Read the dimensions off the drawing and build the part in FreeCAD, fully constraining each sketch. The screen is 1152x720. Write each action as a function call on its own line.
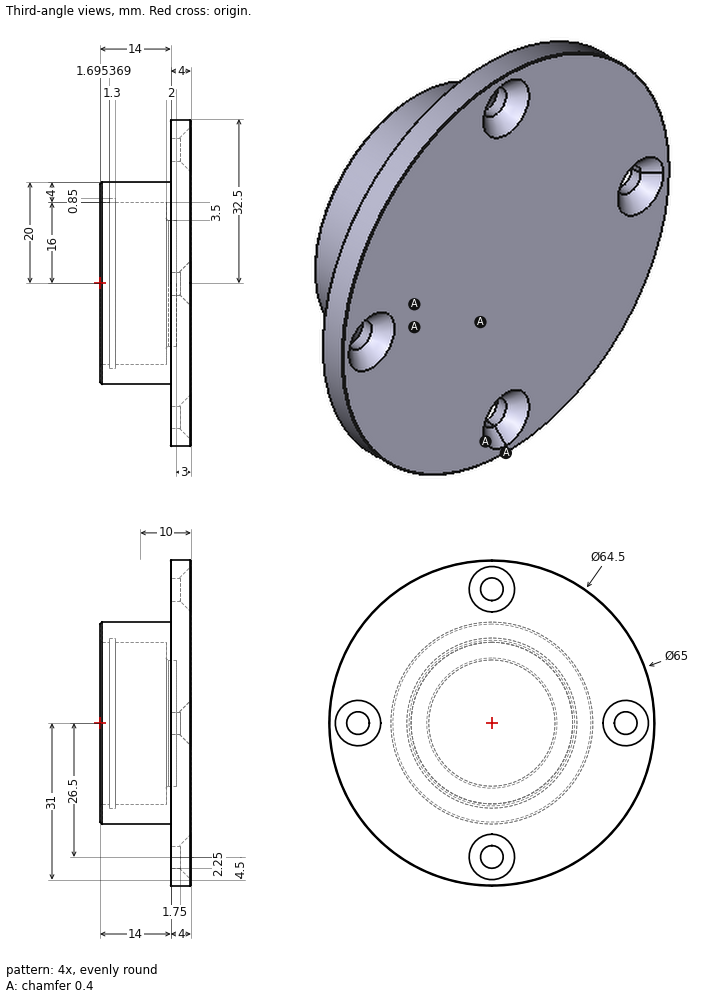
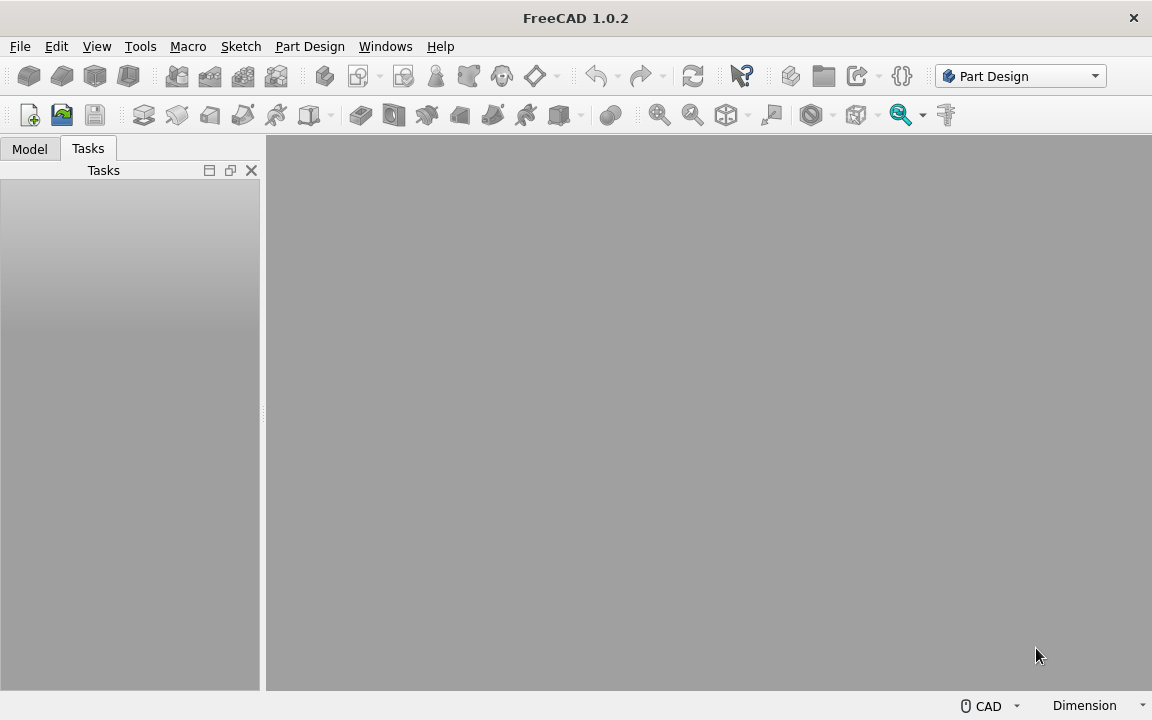
click(29, 116)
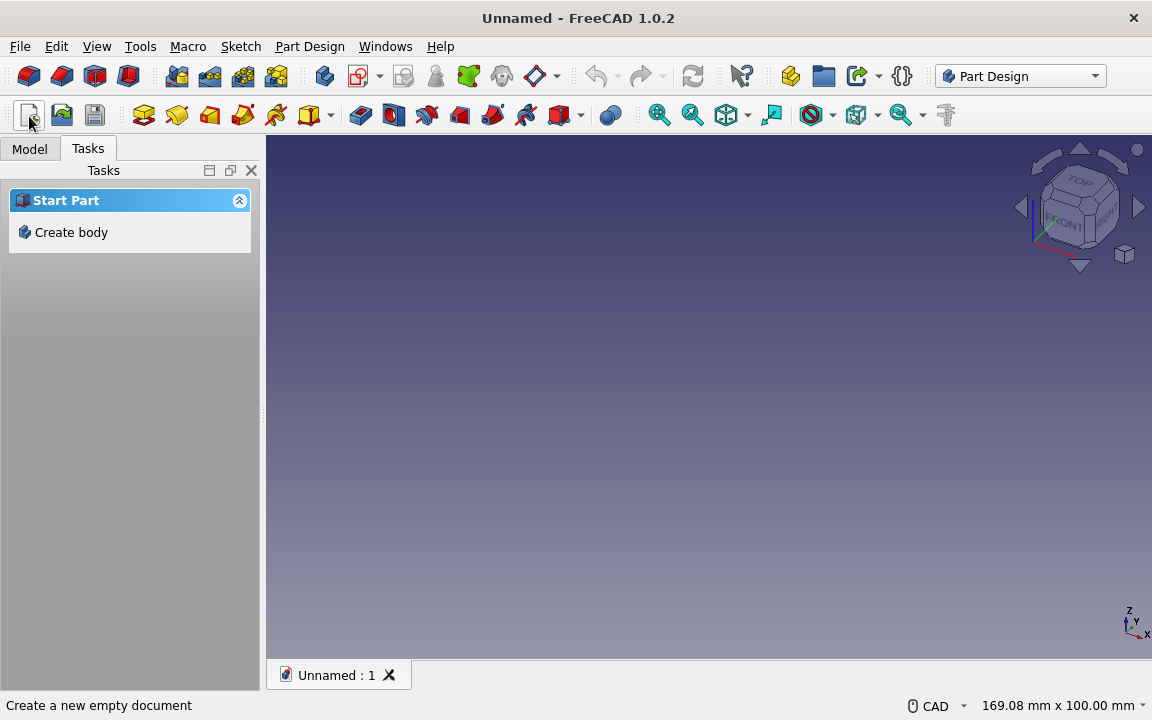
click(358, 76)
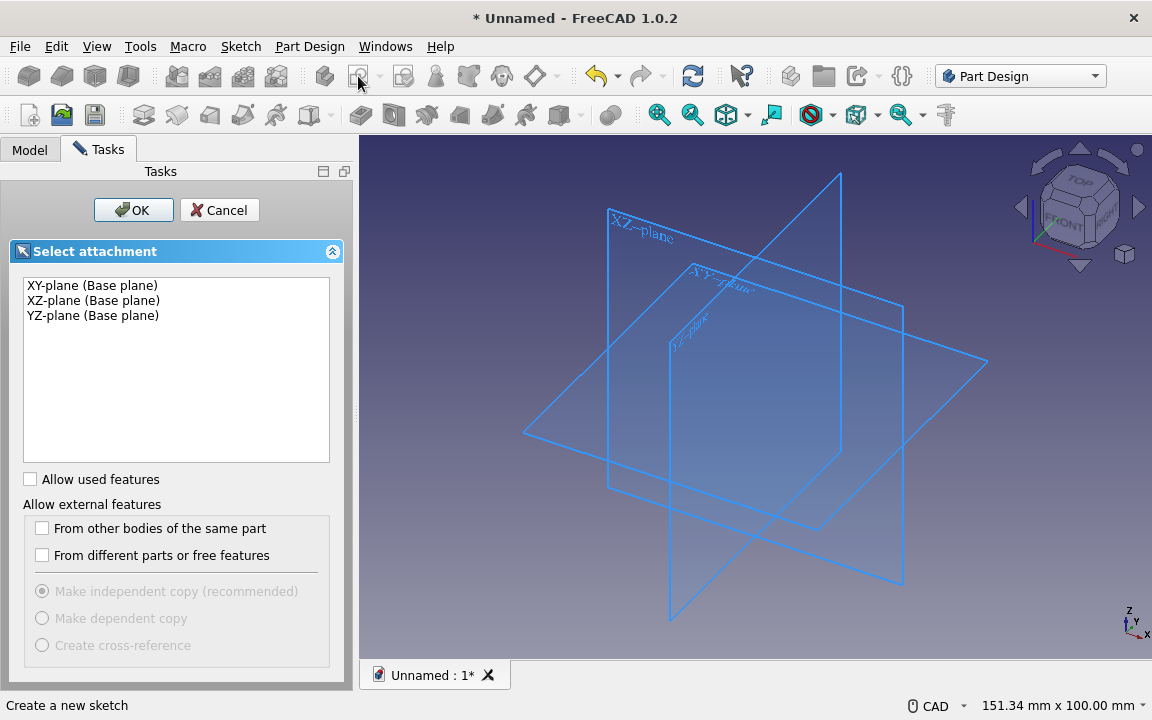
click(84, 286)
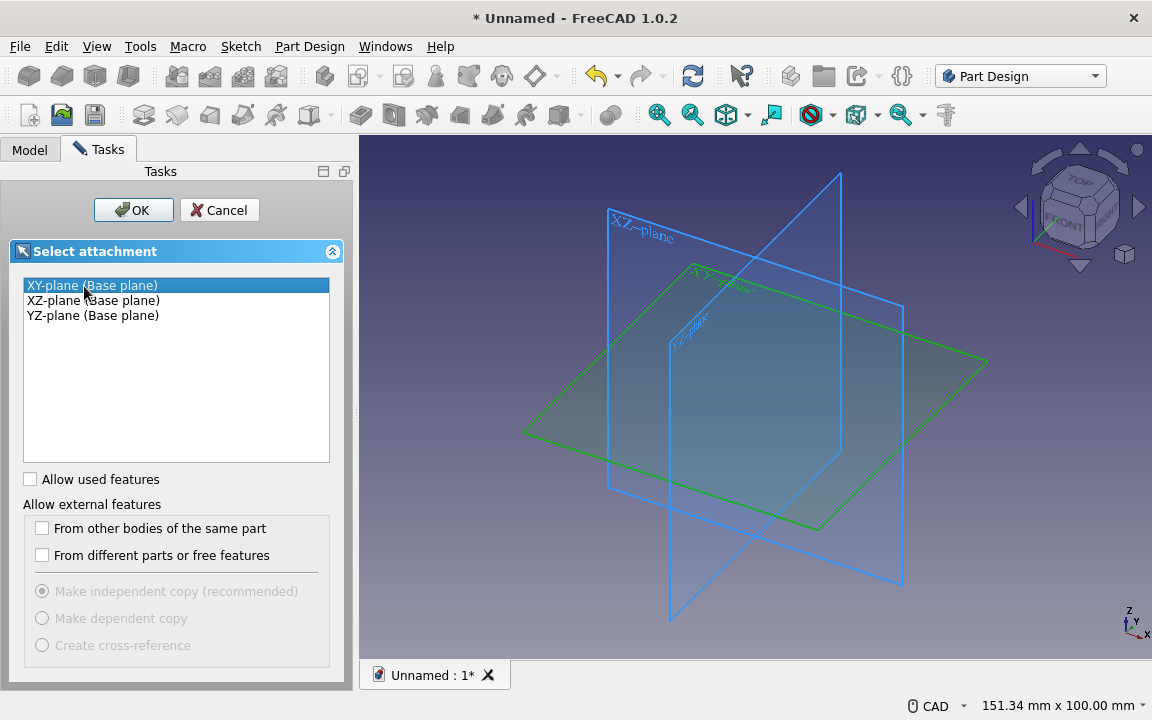
click(134, 210)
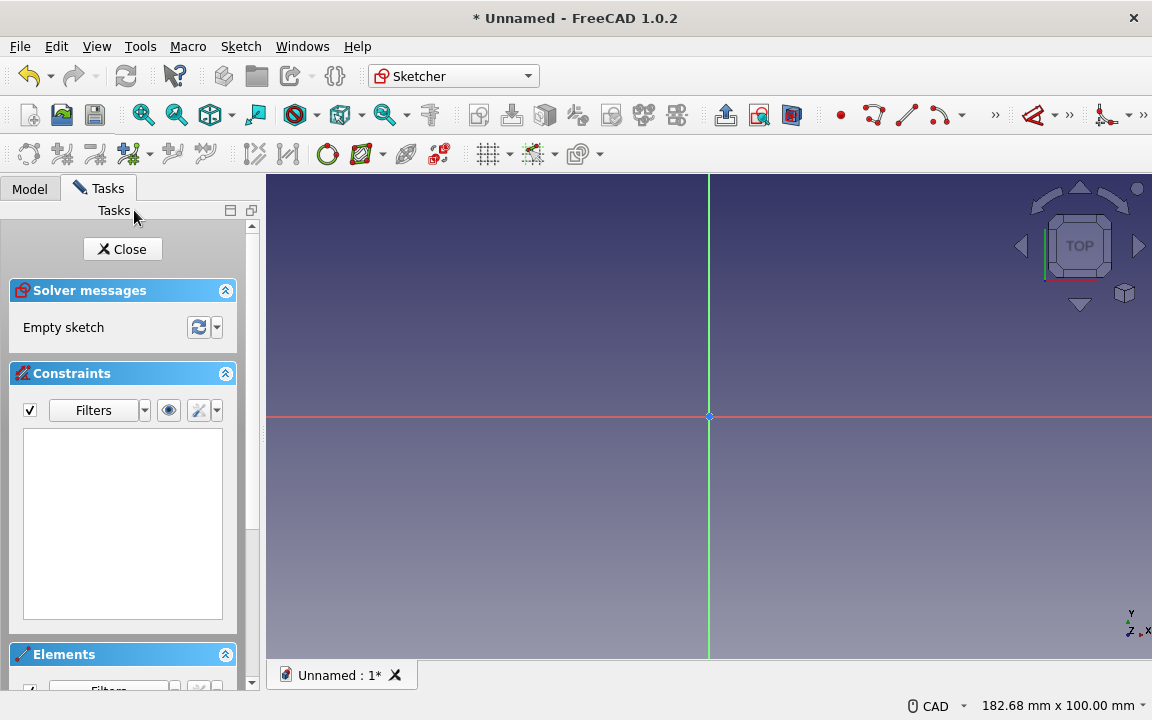
scroll(889, 242, up, 3)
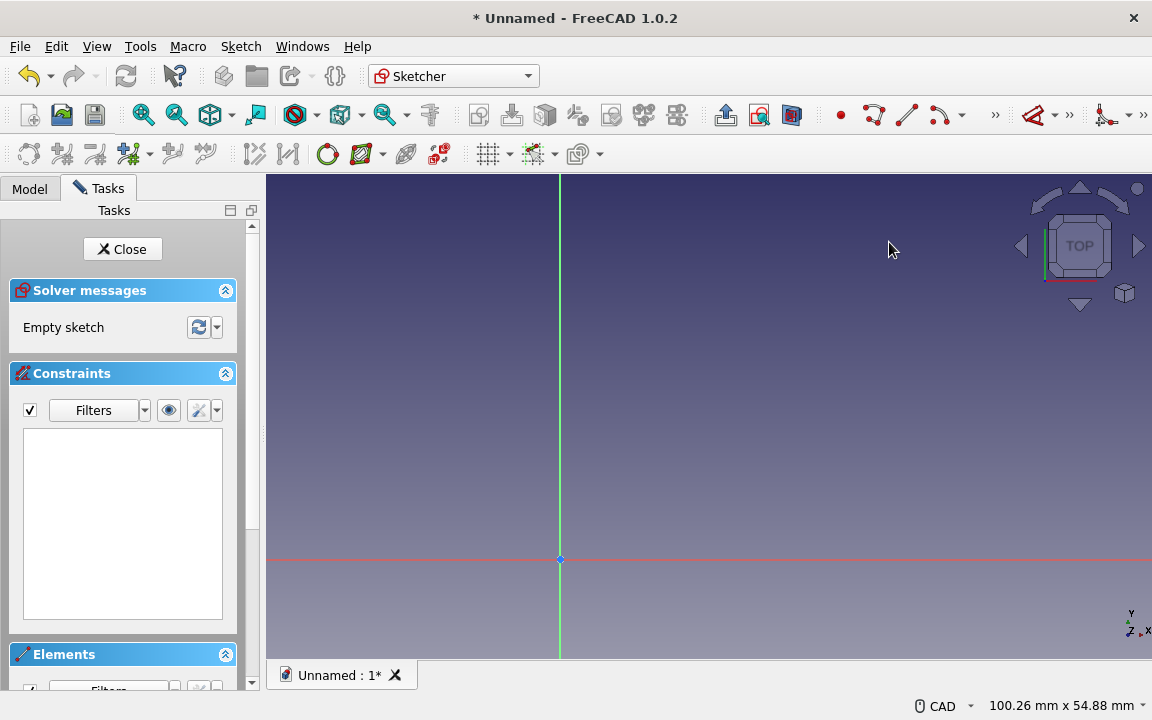
click(874, 116)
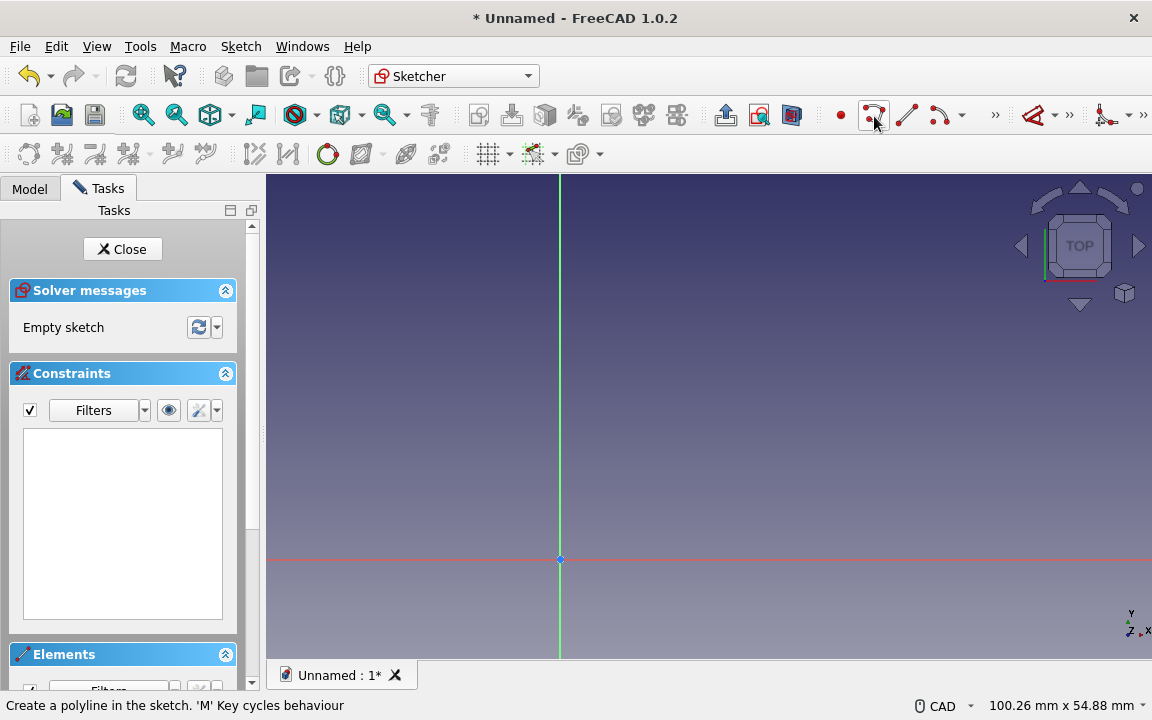
click(693, 560)
click(720, 551)
click(720, 273)
click(684, 273)
click(684, 383)
click(560, 383)
click(569, 418)
click(575, 418)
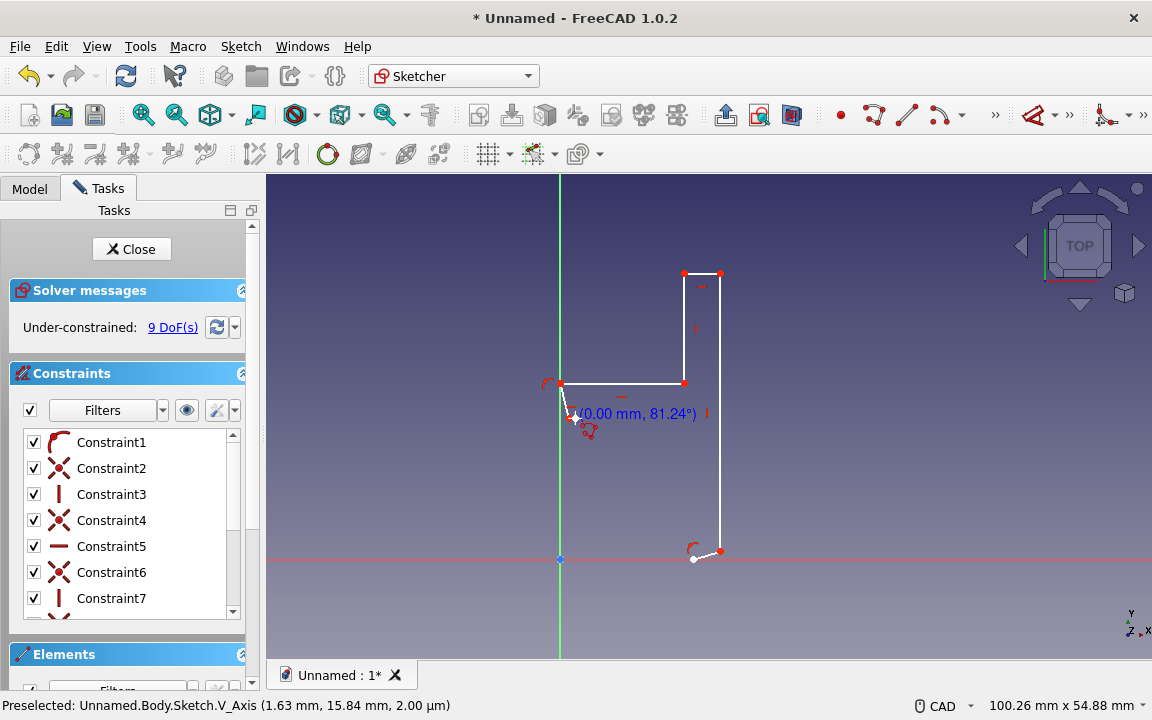
scroll(575, 411, up, 4)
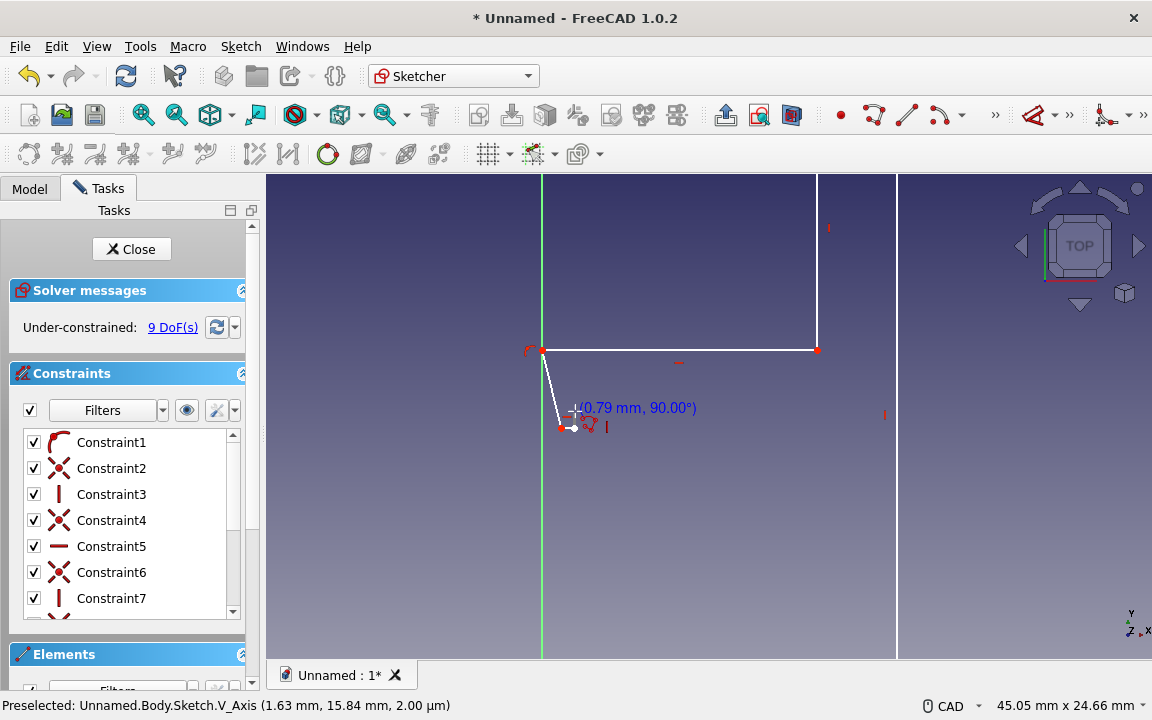
click(575, 410)
click(601, 410)
click(601, 427)
click(798, 427)
click(798, 496)
click(837, 496)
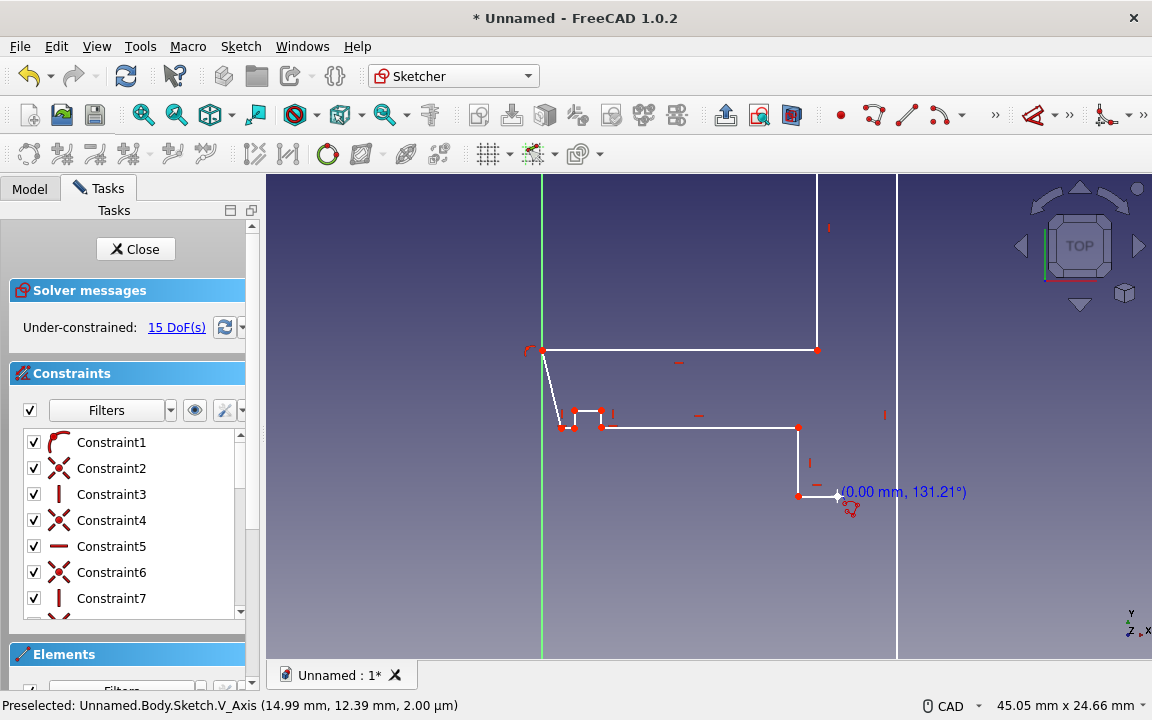
scroll(576, 412, down, 4)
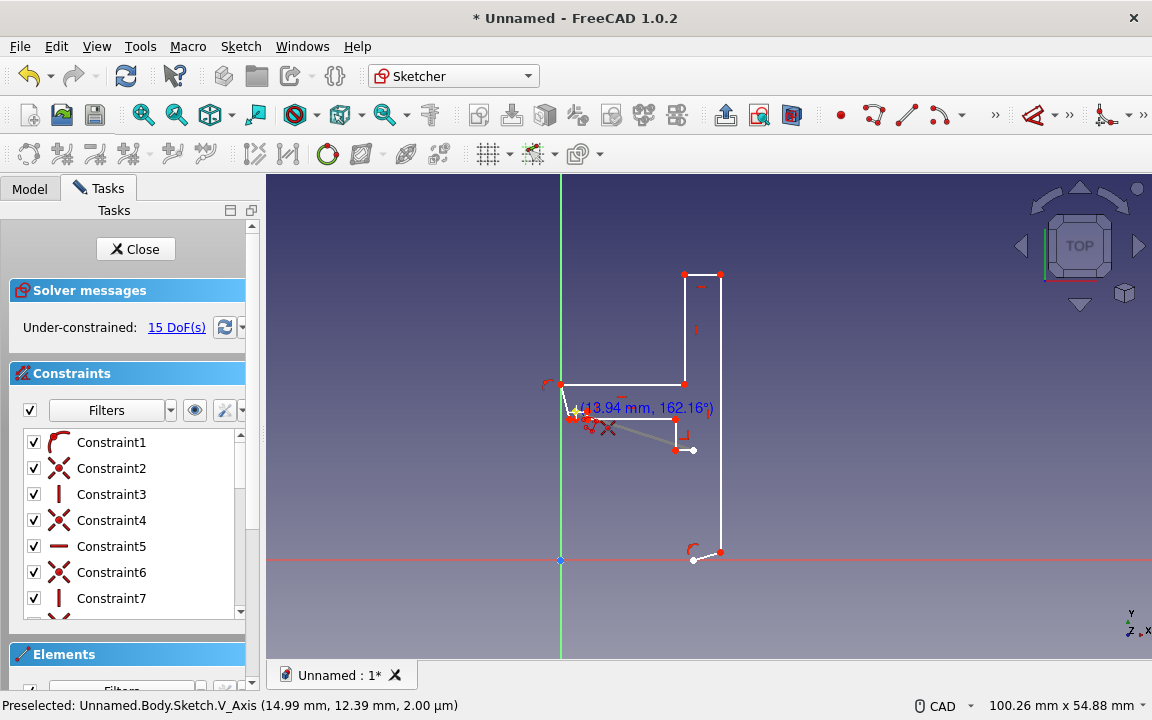
click(694, 560)
key(Escape)
key(Escape)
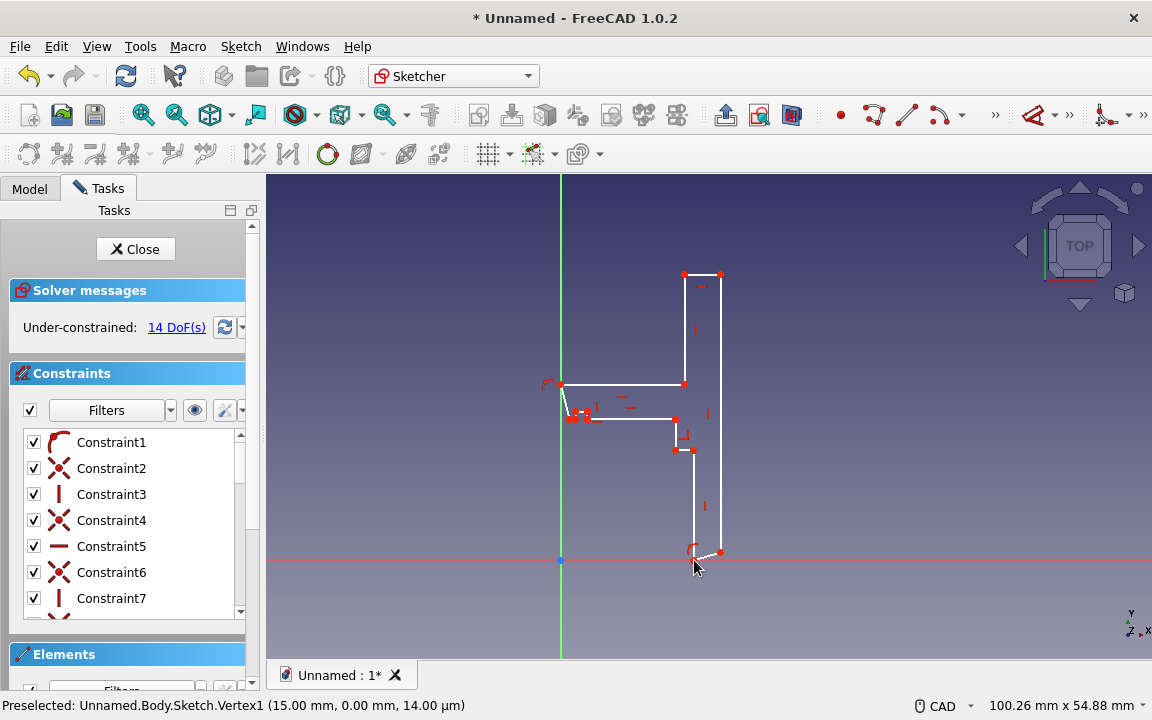
scroll(704, 557, up, 2)